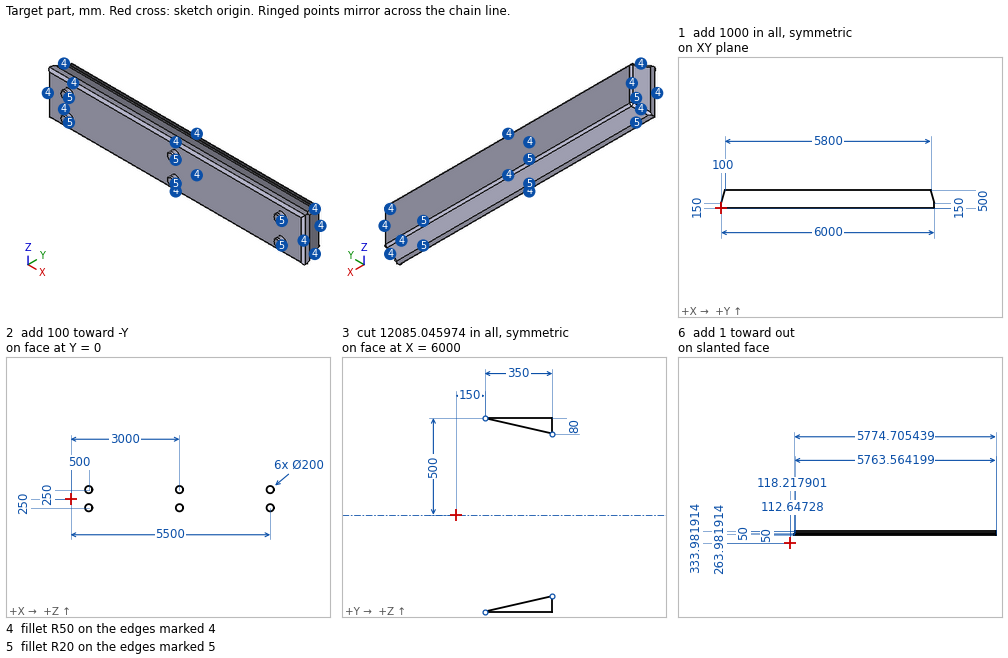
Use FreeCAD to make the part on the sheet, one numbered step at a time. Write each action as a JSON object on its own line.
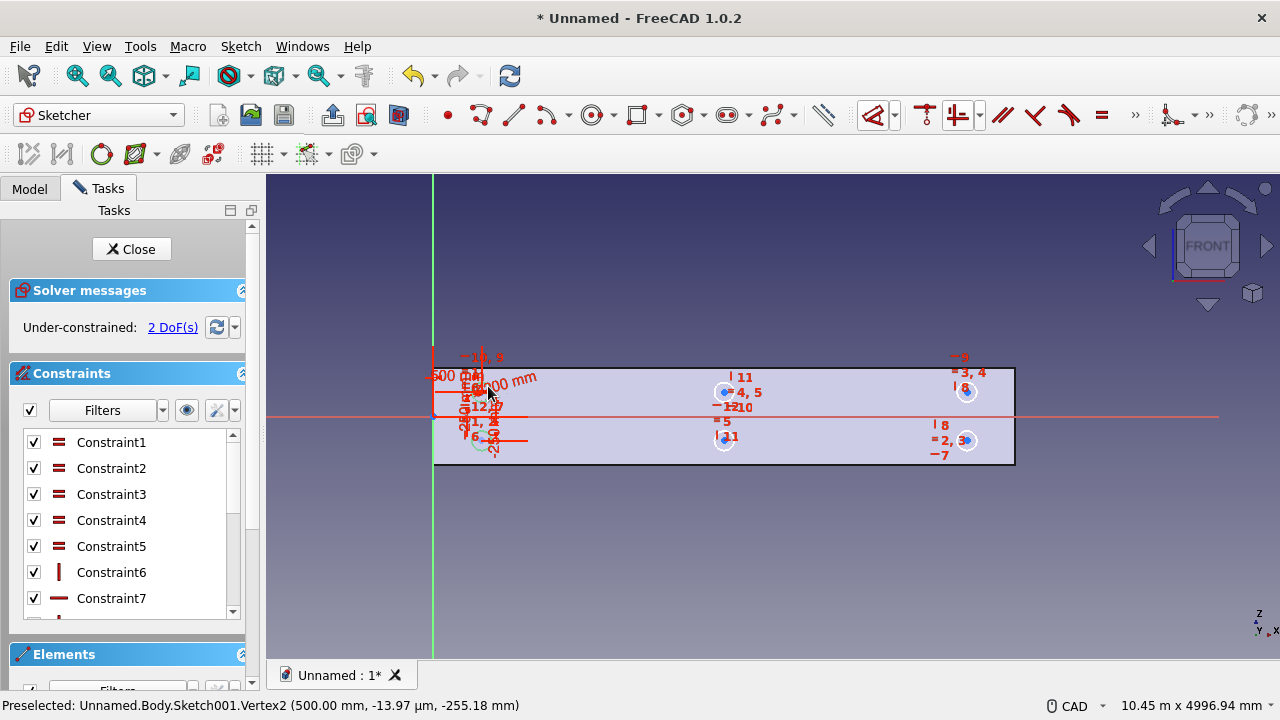
{"action": "left_click", "coordinate": [967, 441]}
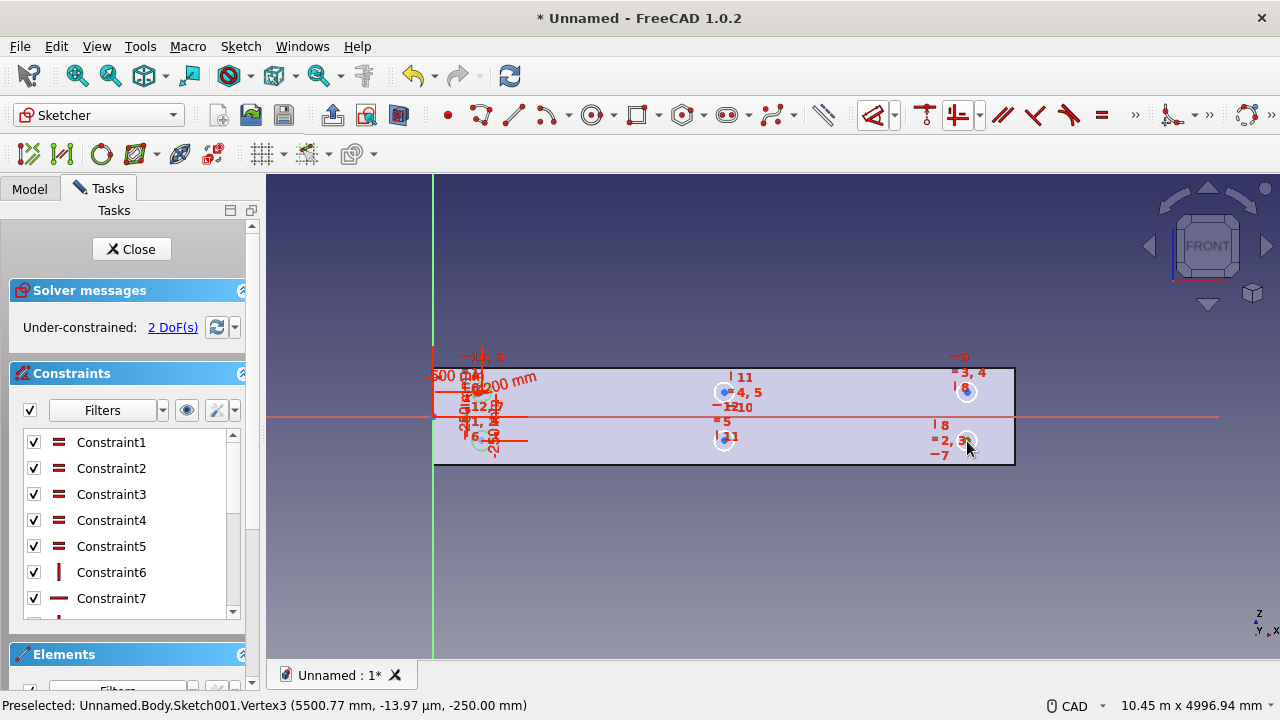
{"action": "left_click", "coordinate": [894, 116]}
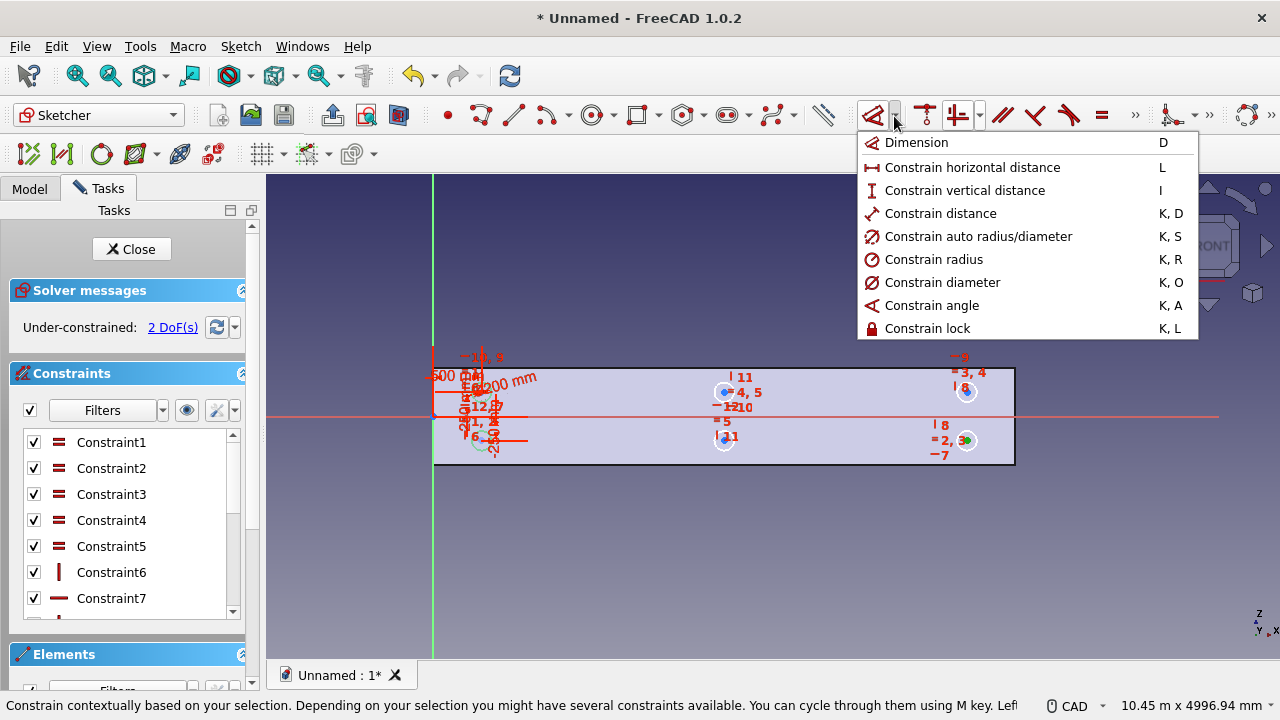
{"action": "left_click", "coordinate": [1028, 168]}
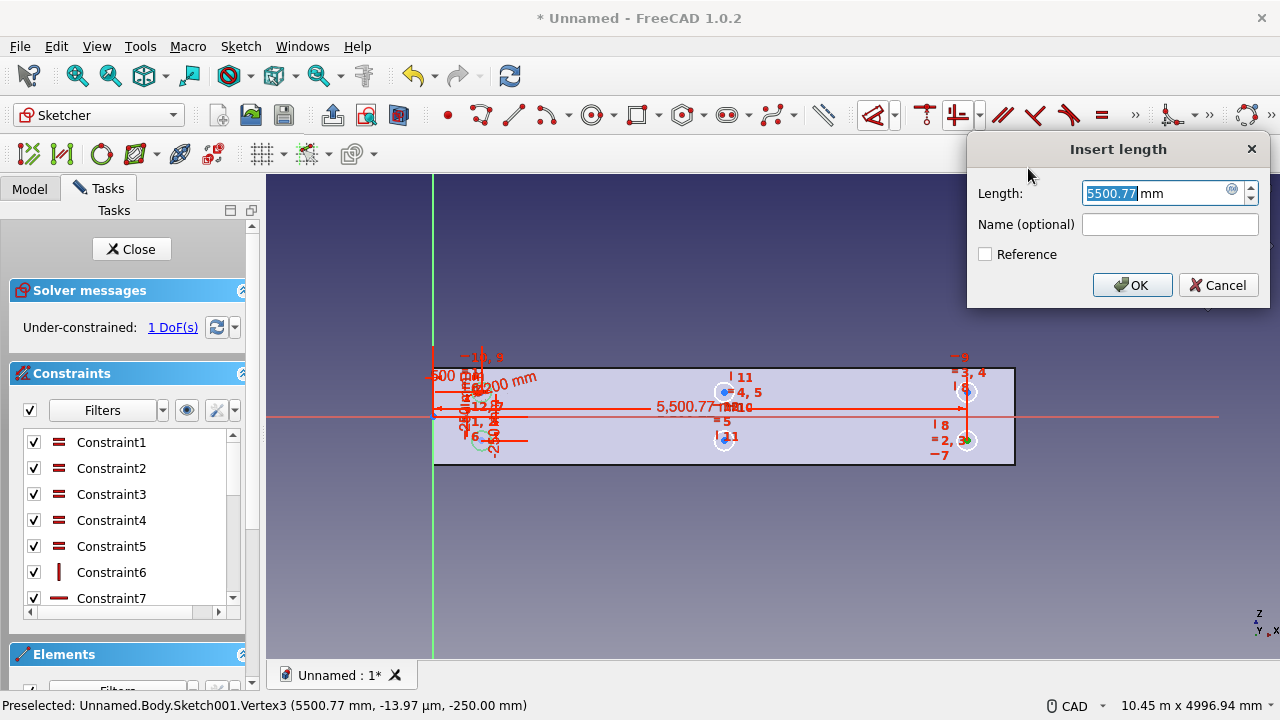
{"action": "type", "text": "5500"}
{"action": "key", "text": "Return"}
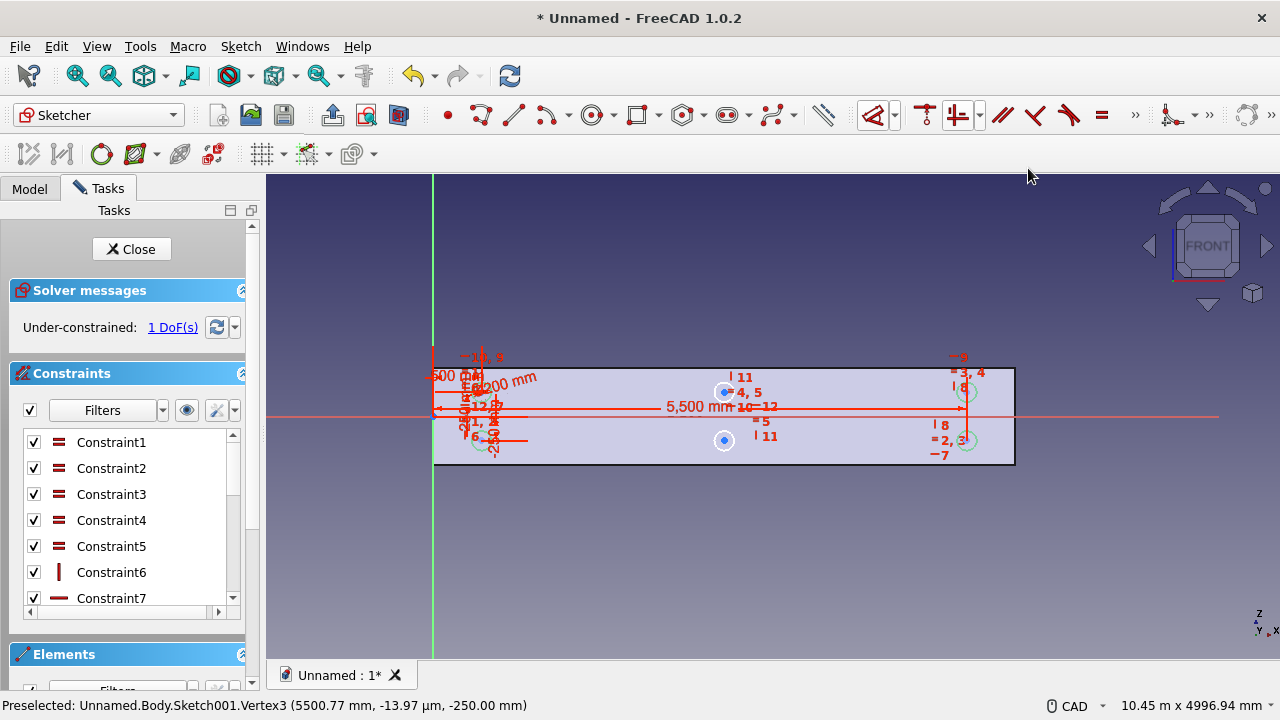
{"action": "left_click", "coordinate": [724, 392]}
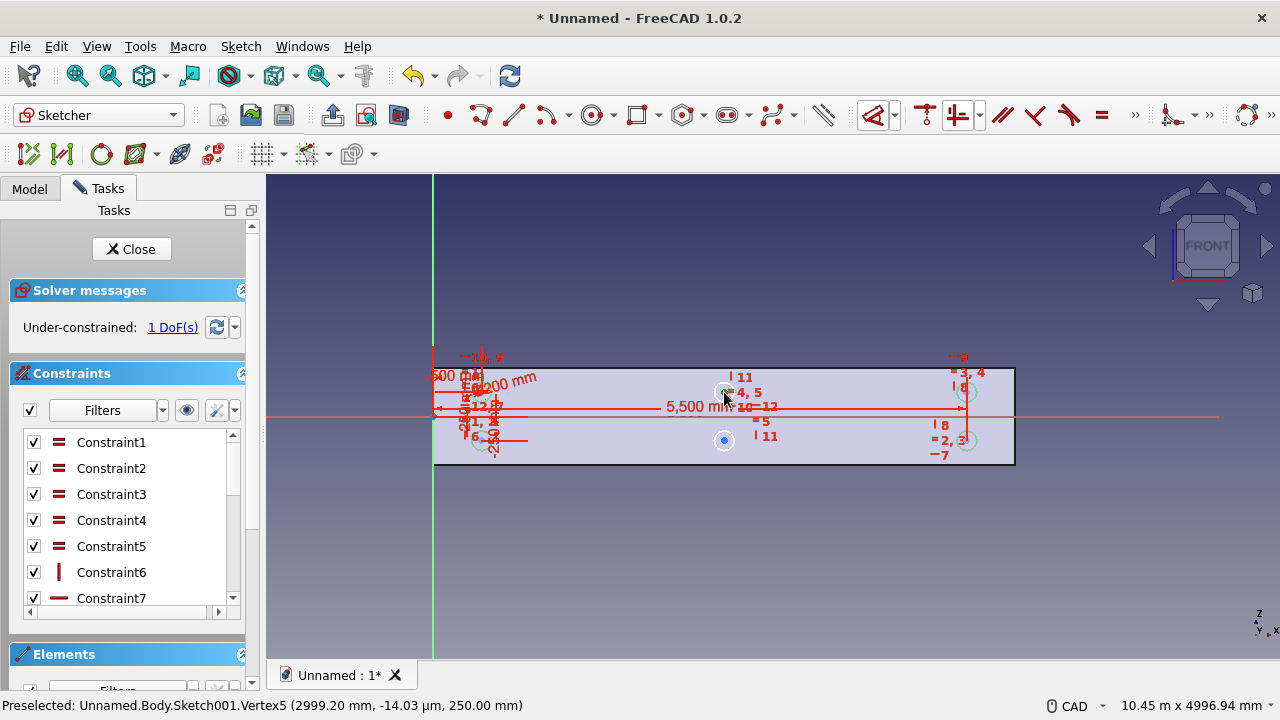
{"action": "key", "text": "l"}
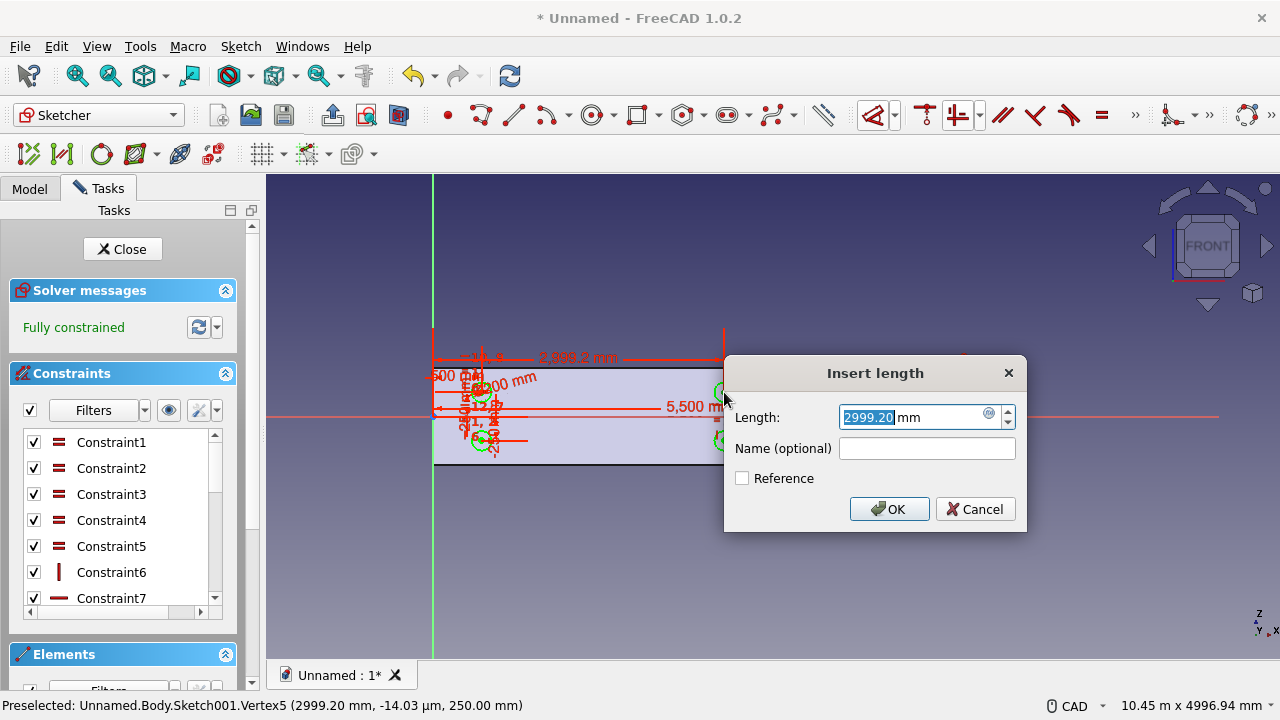
{"action": "type", "text": "3000"}
{"action": "key", "text": "Return"}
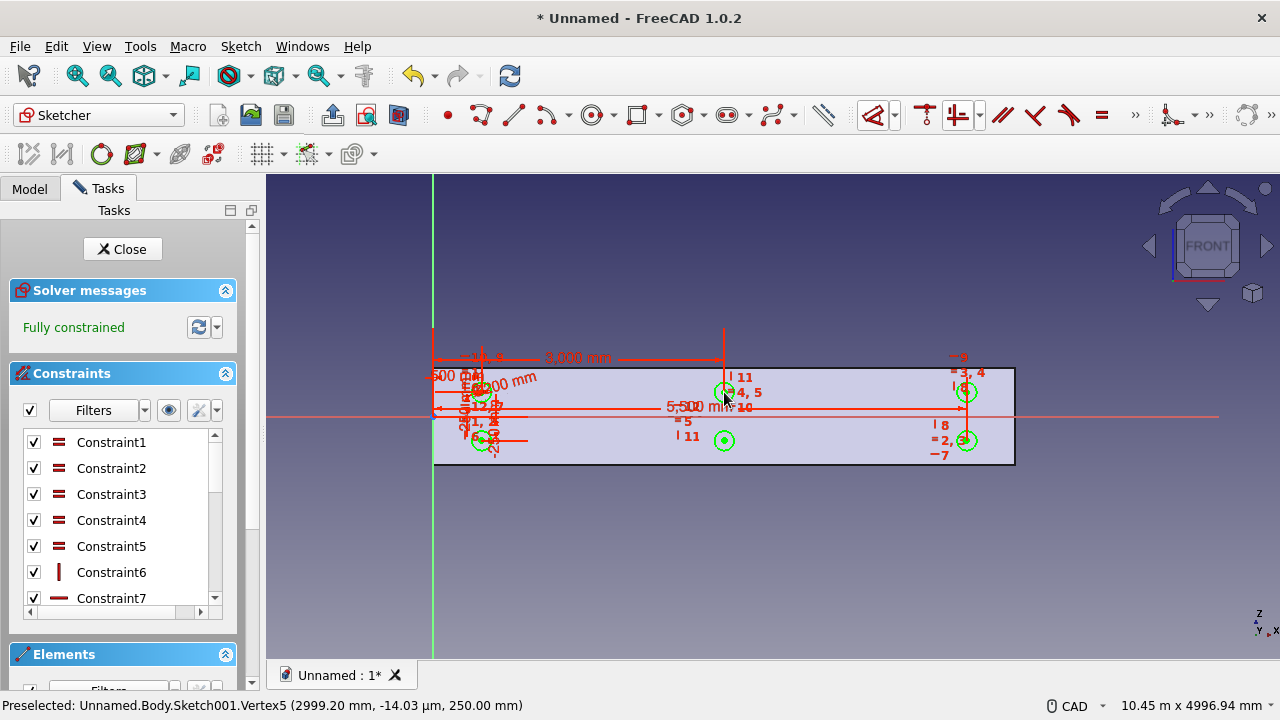
{"action": "left_click", "coordinate": [123, 249]}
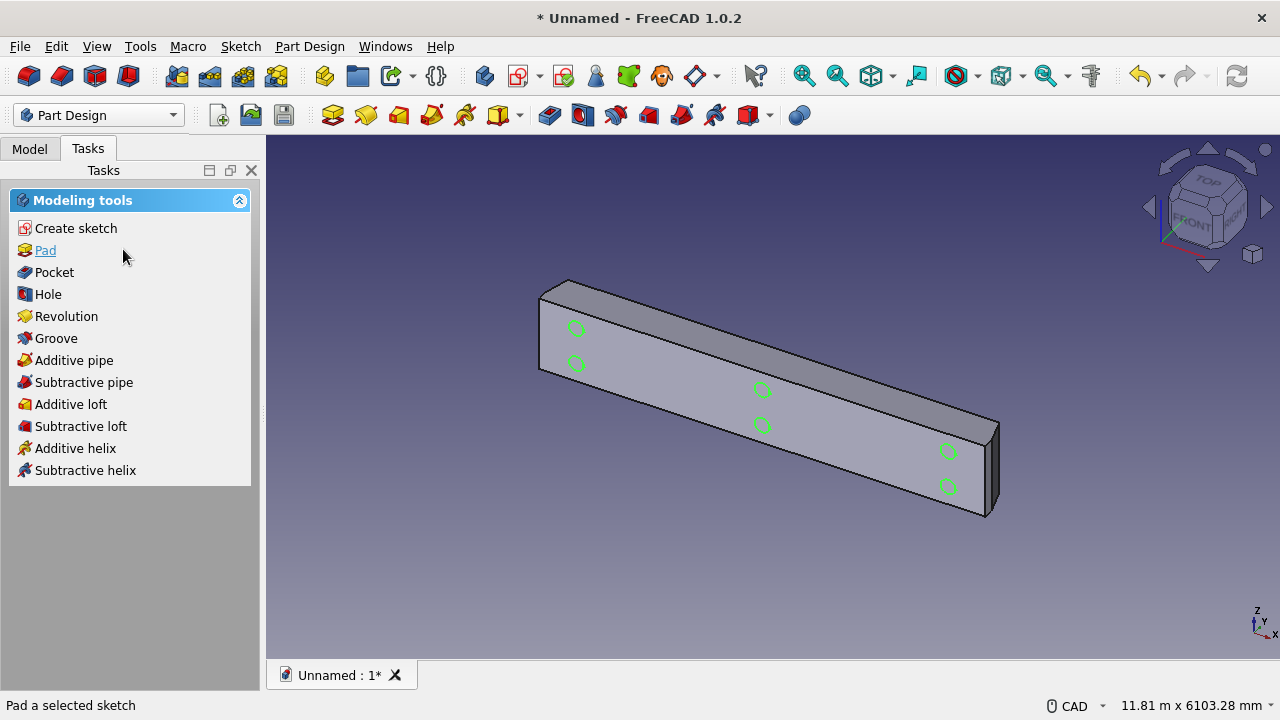
{"action": "left_click", "coordinate": [333, 116]}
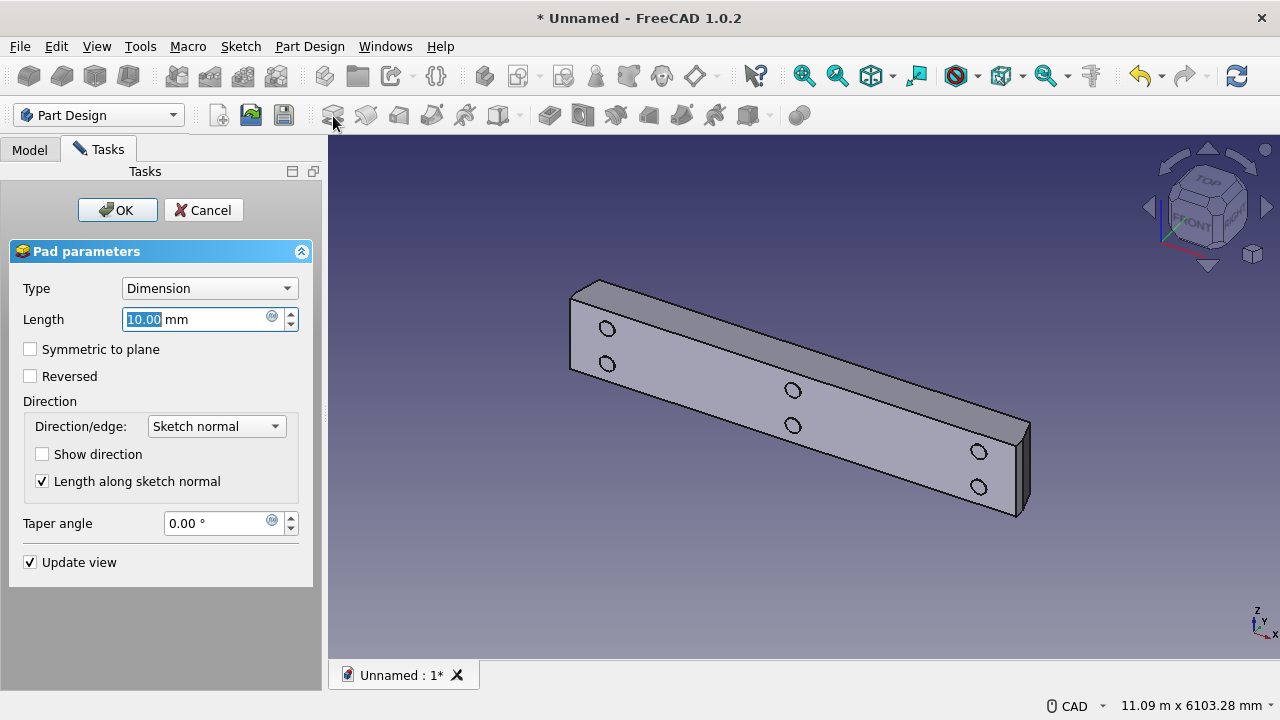
{"action": "type", "text": "100"}
{"action": "key", "text": "Tab"}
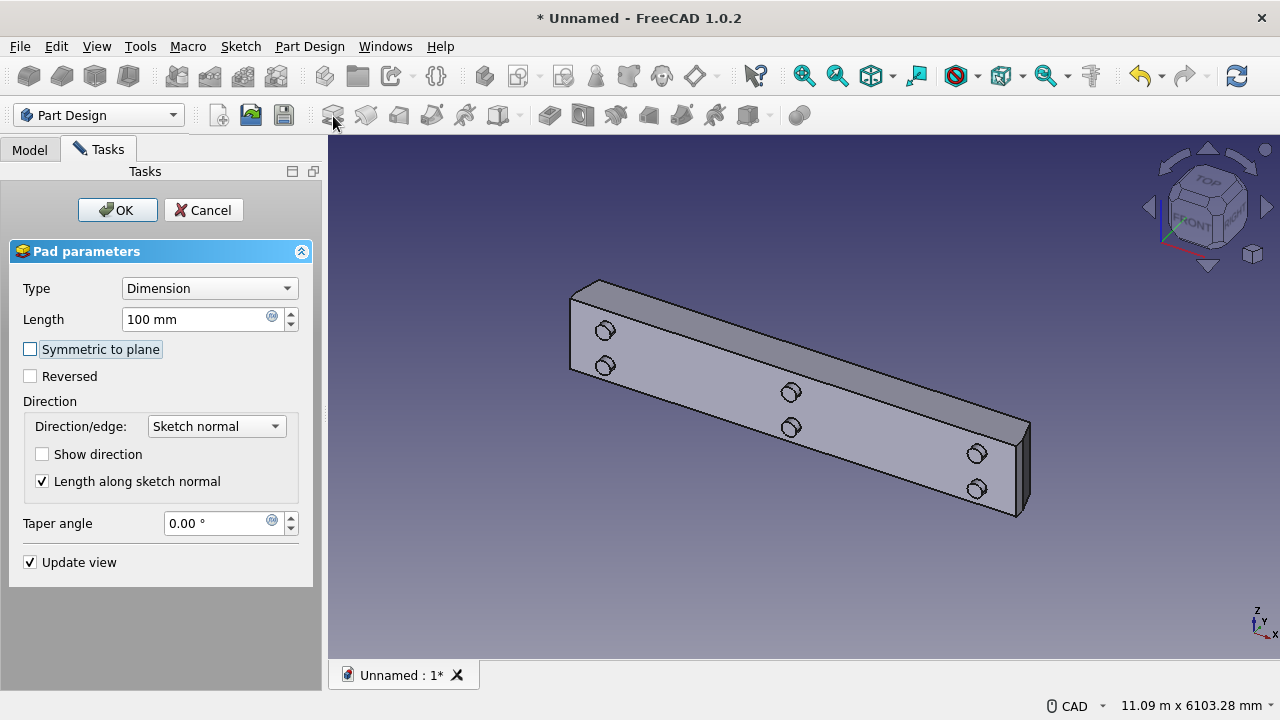
{"action": "left_click", "coordinate": [118, 210]}